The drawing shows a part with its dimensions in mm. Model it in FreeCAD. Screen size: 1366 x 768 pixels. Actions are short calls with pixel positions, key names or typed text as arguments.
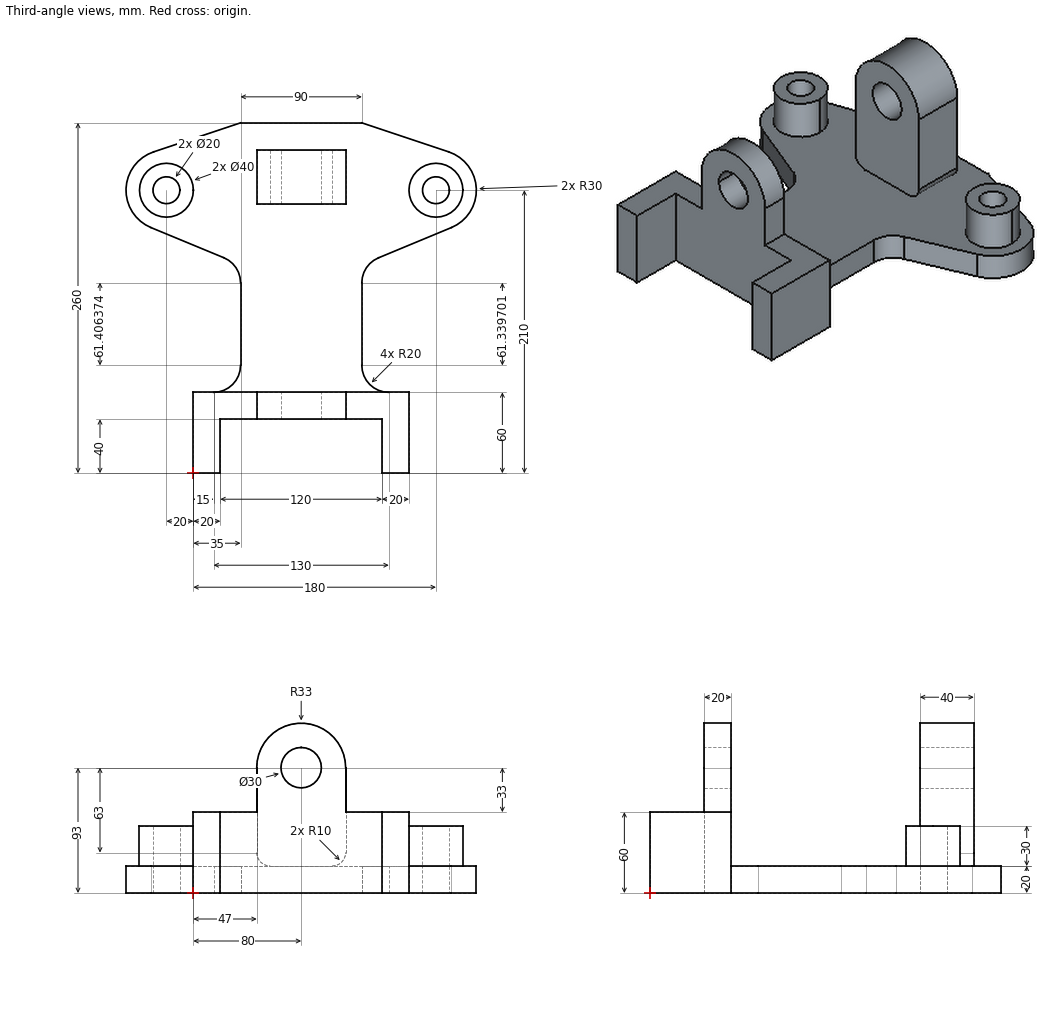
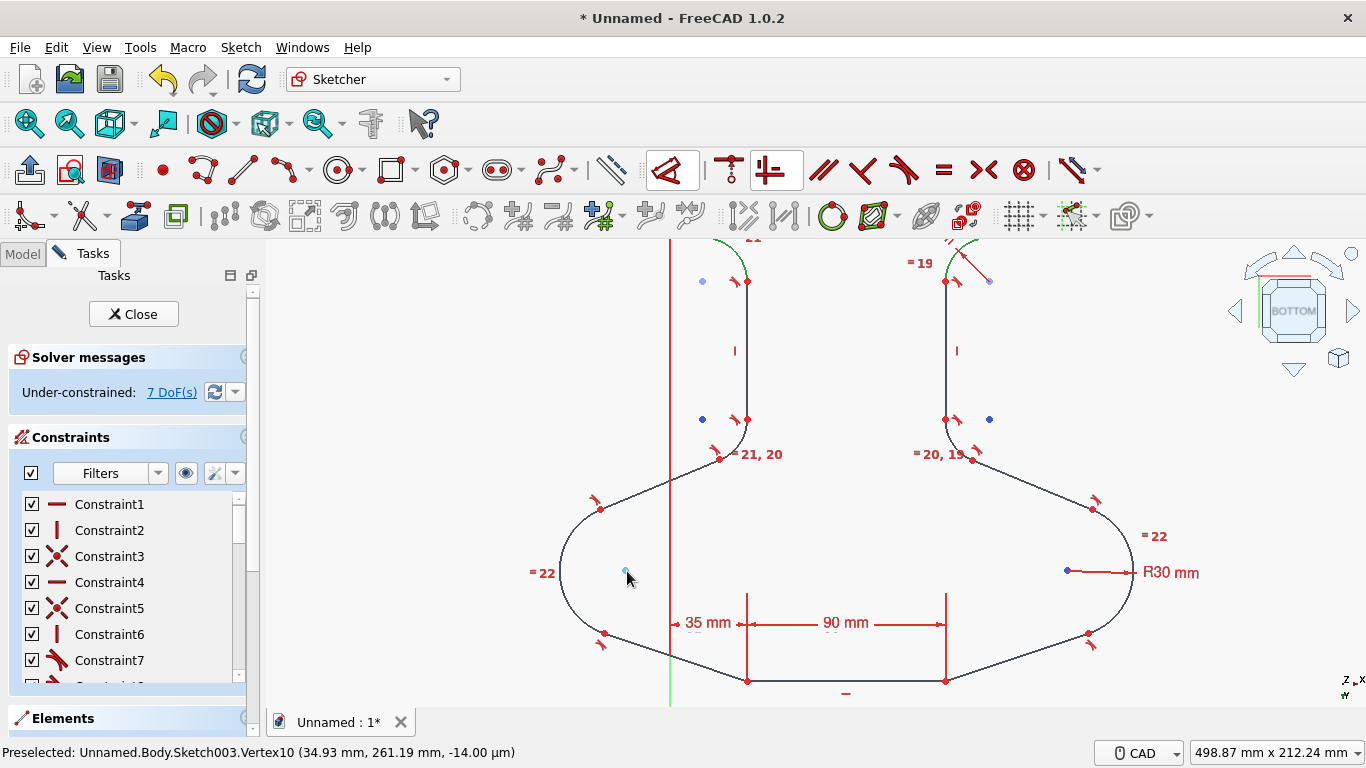
click(626, 571)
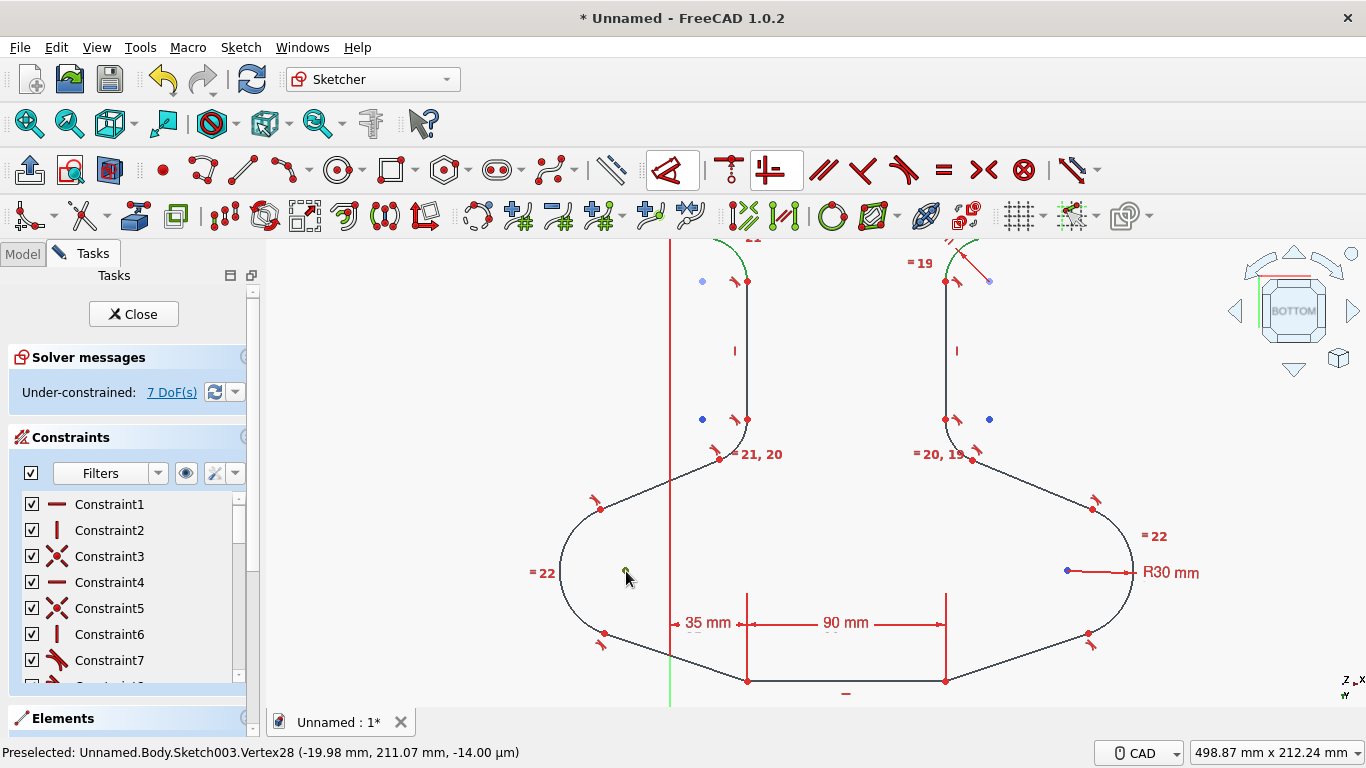
click(694, 170)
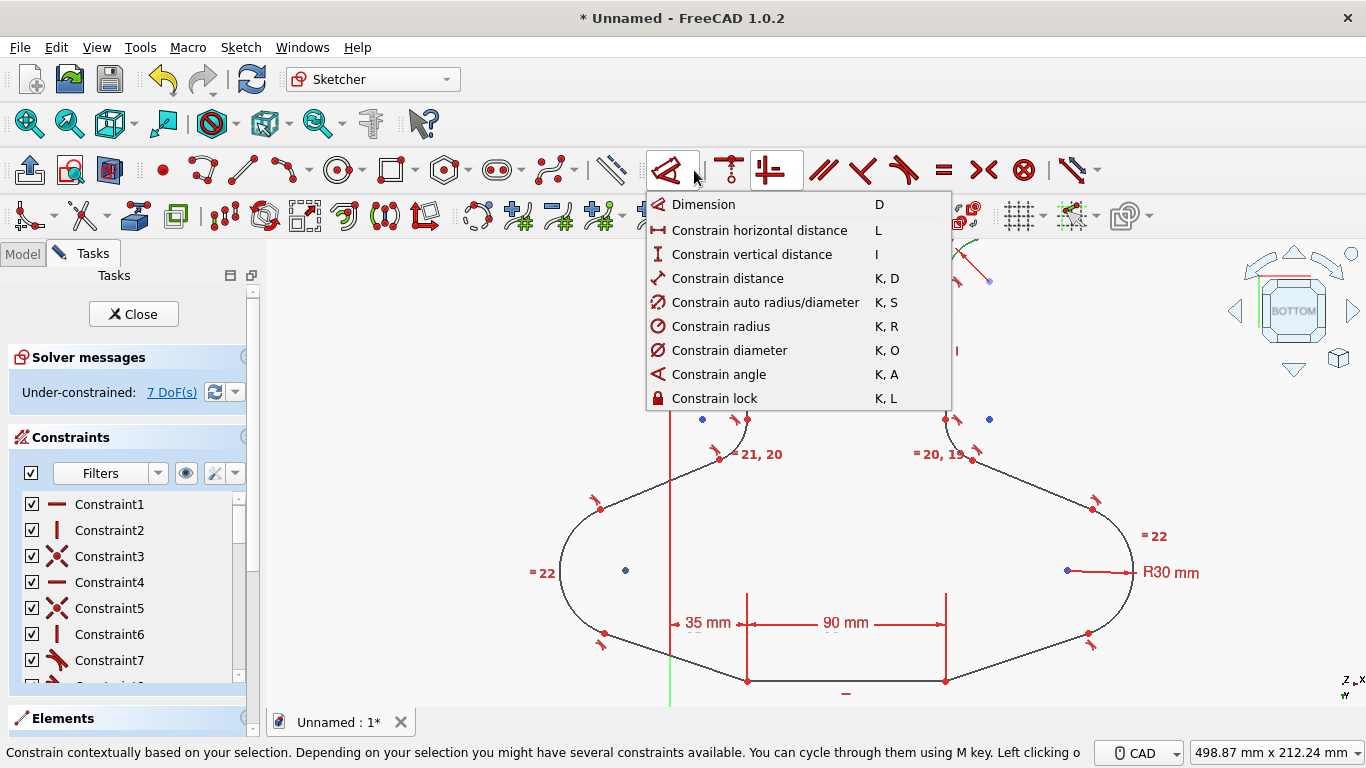
click(799, 230)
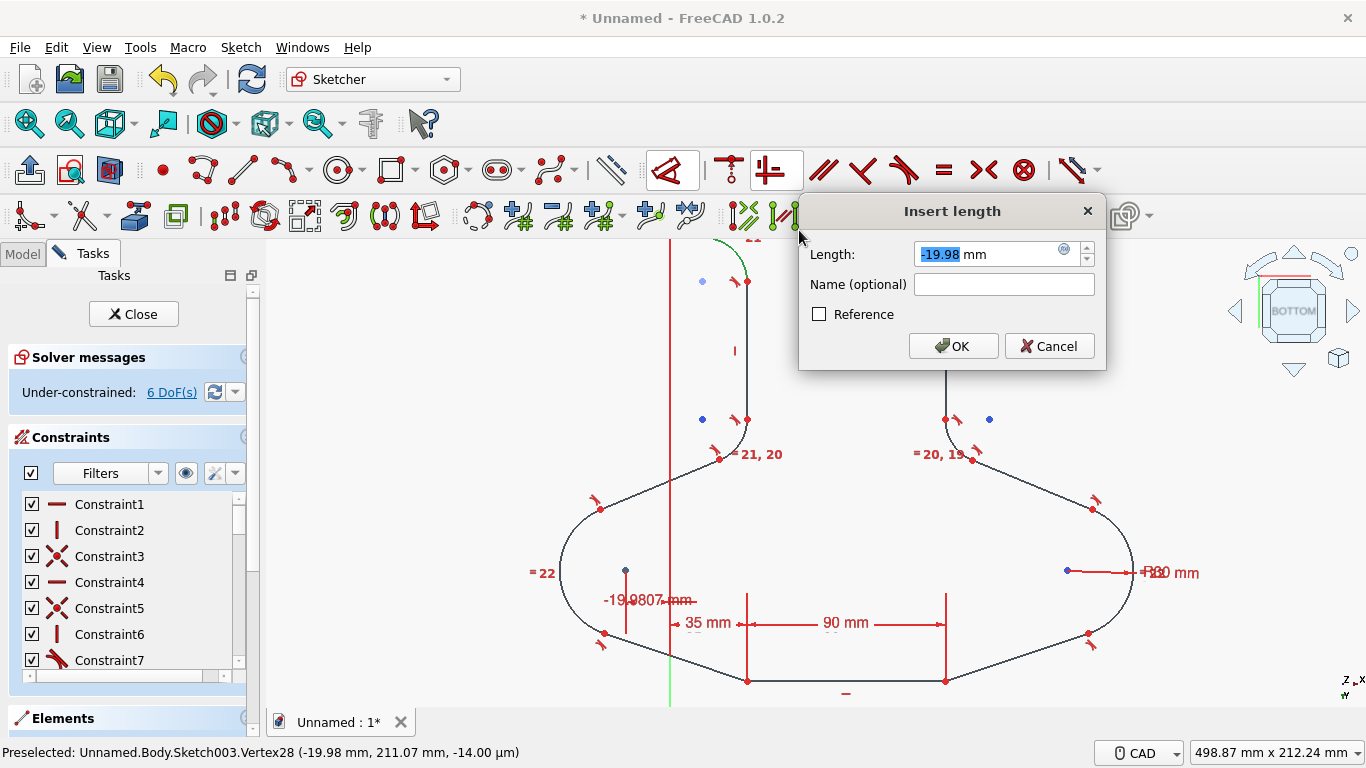
text(-20)
key(Return)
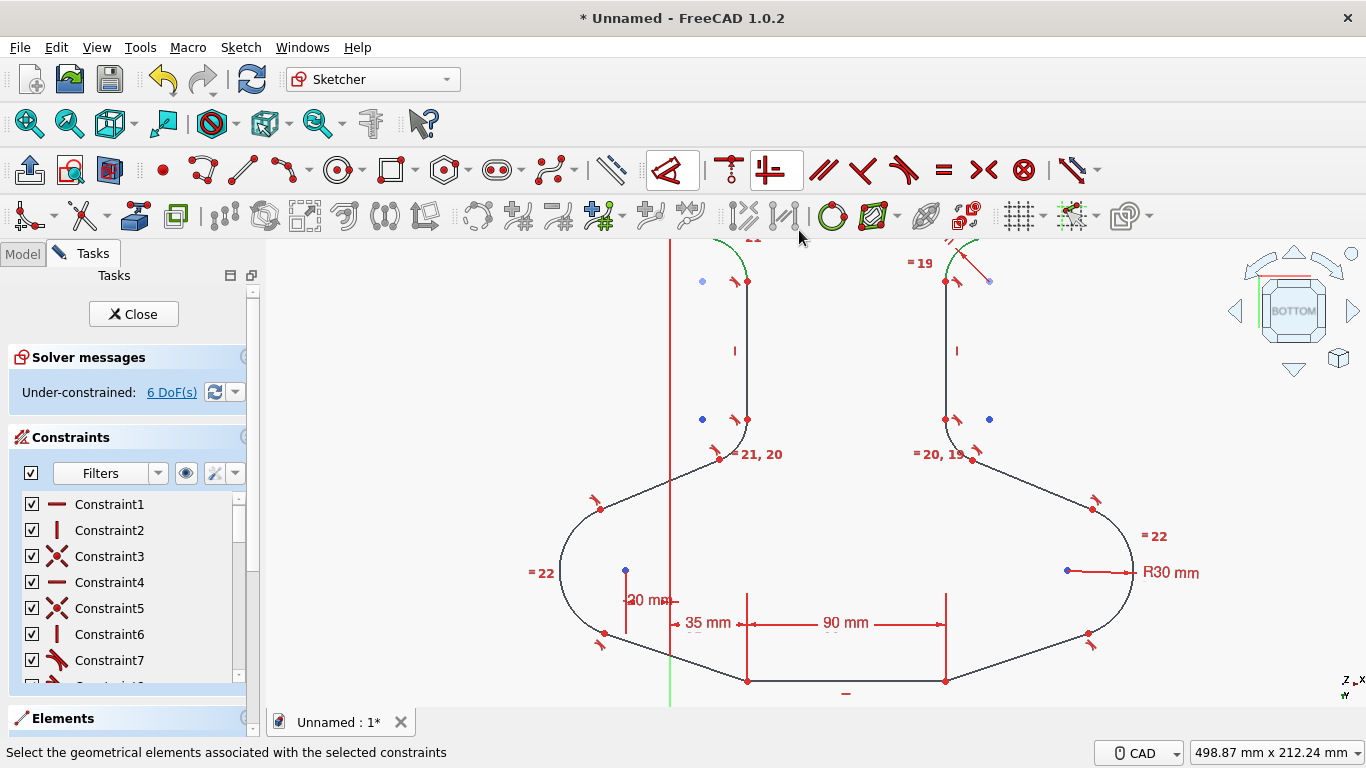
scroll(627, 571, down, 3)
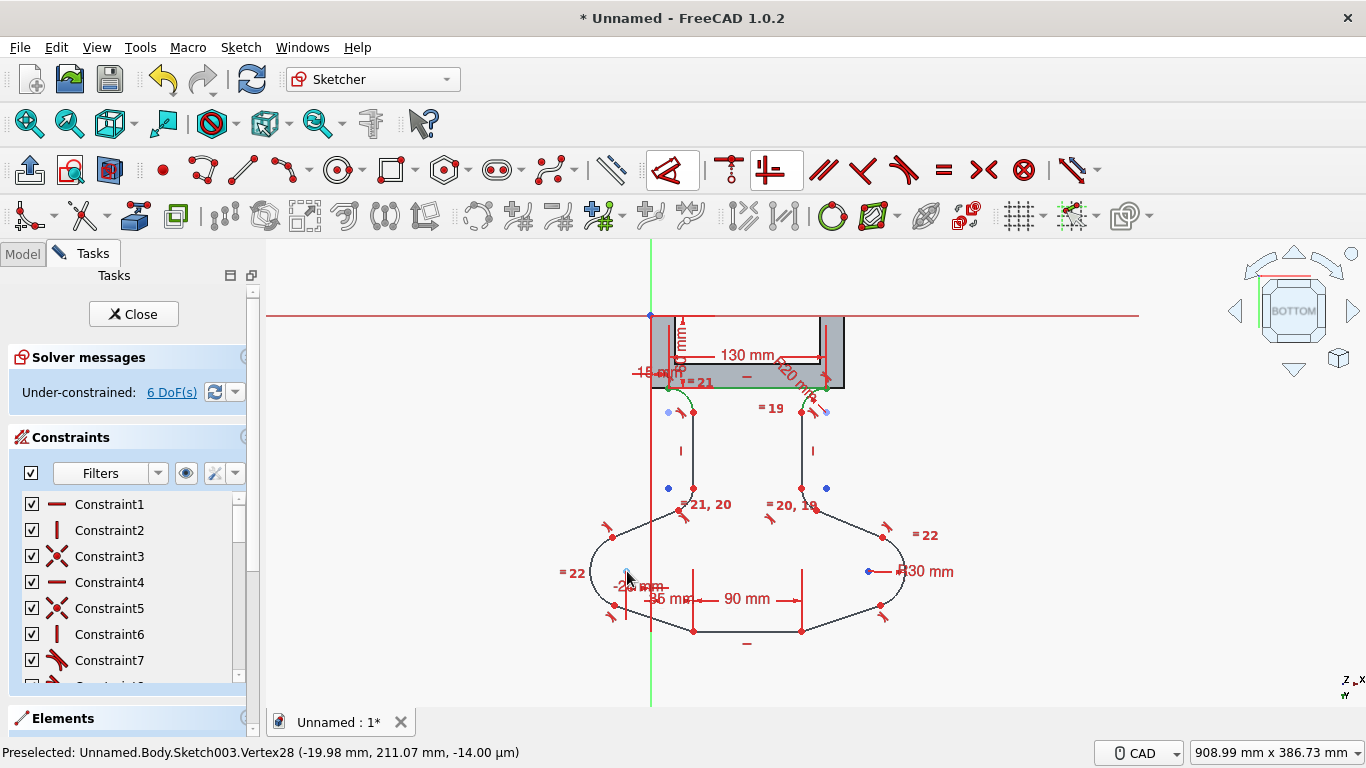
click(802, 632)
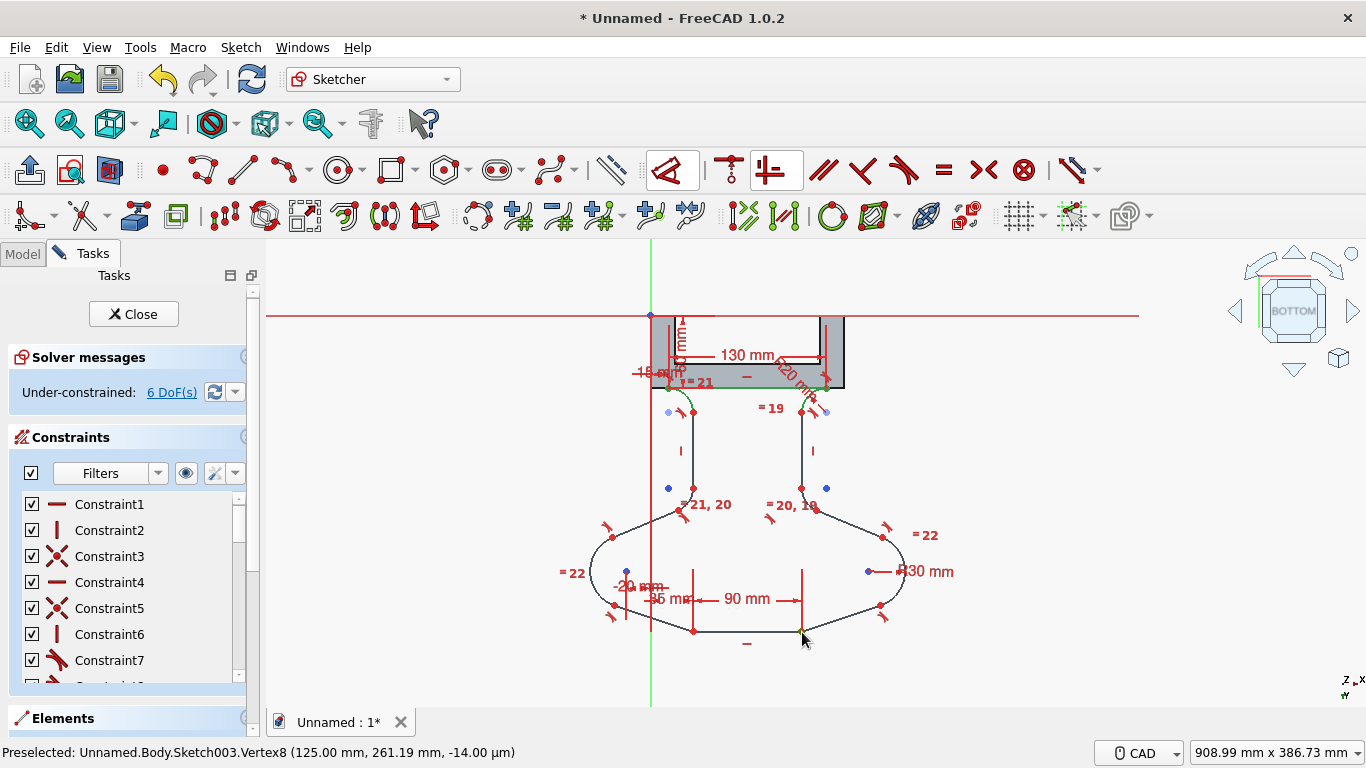
click(694, 170)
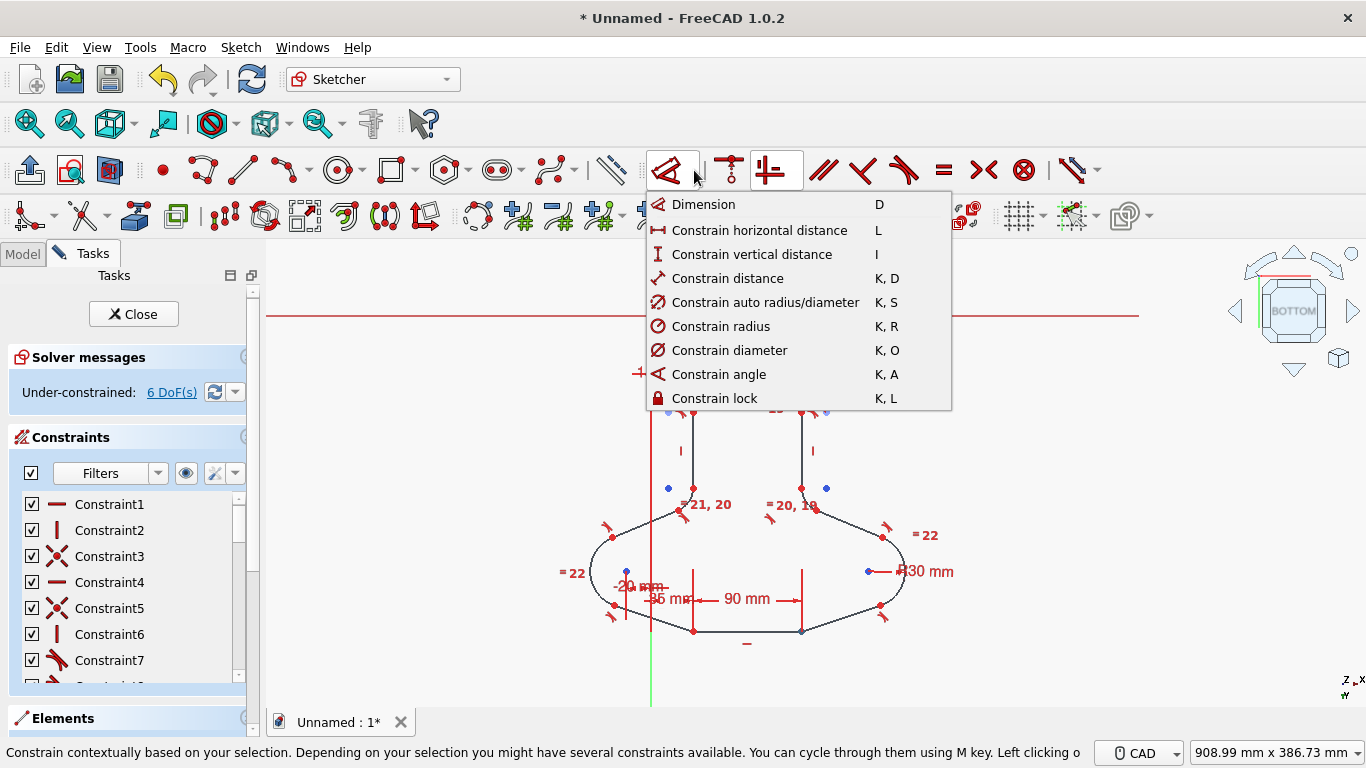
click(799, 254)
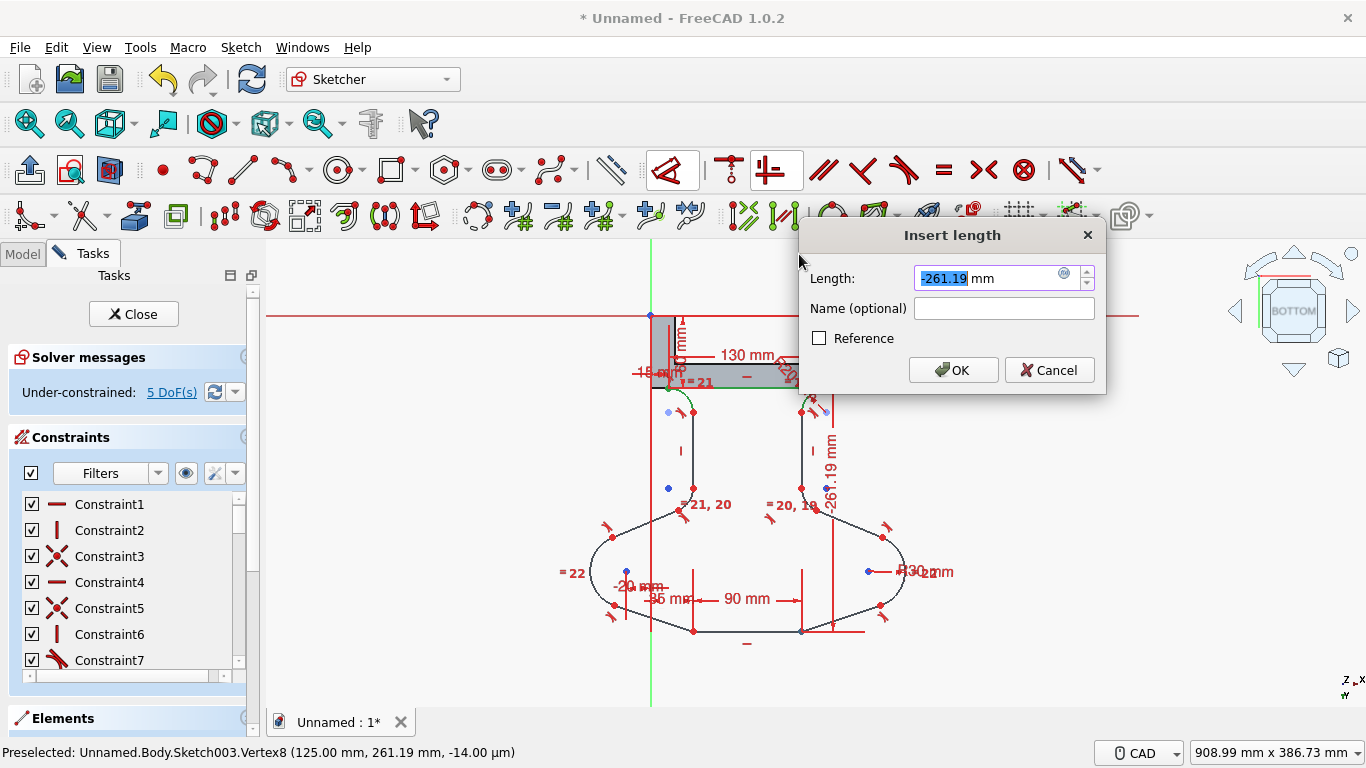
text(-260)
key(Return)